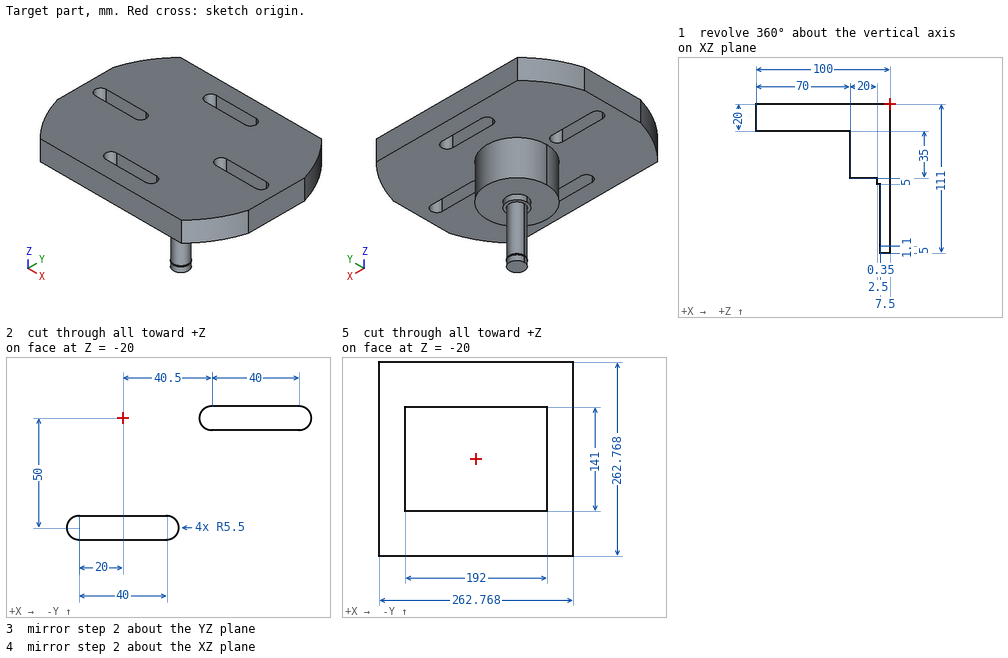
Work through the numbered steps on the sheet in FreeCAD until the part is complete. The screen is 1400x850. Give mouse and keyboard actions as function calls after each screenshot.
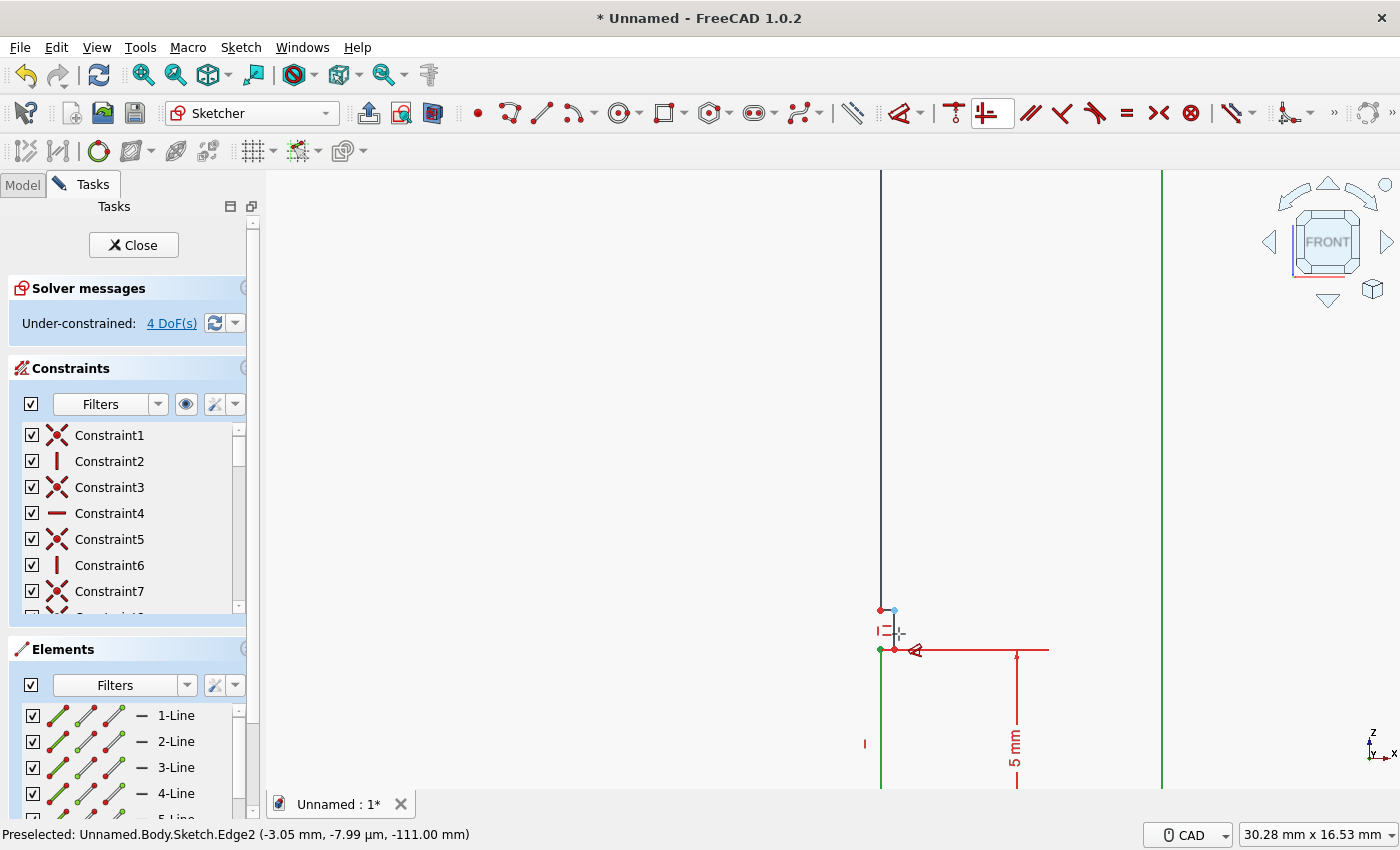
click(894, 630)
click(928, 630)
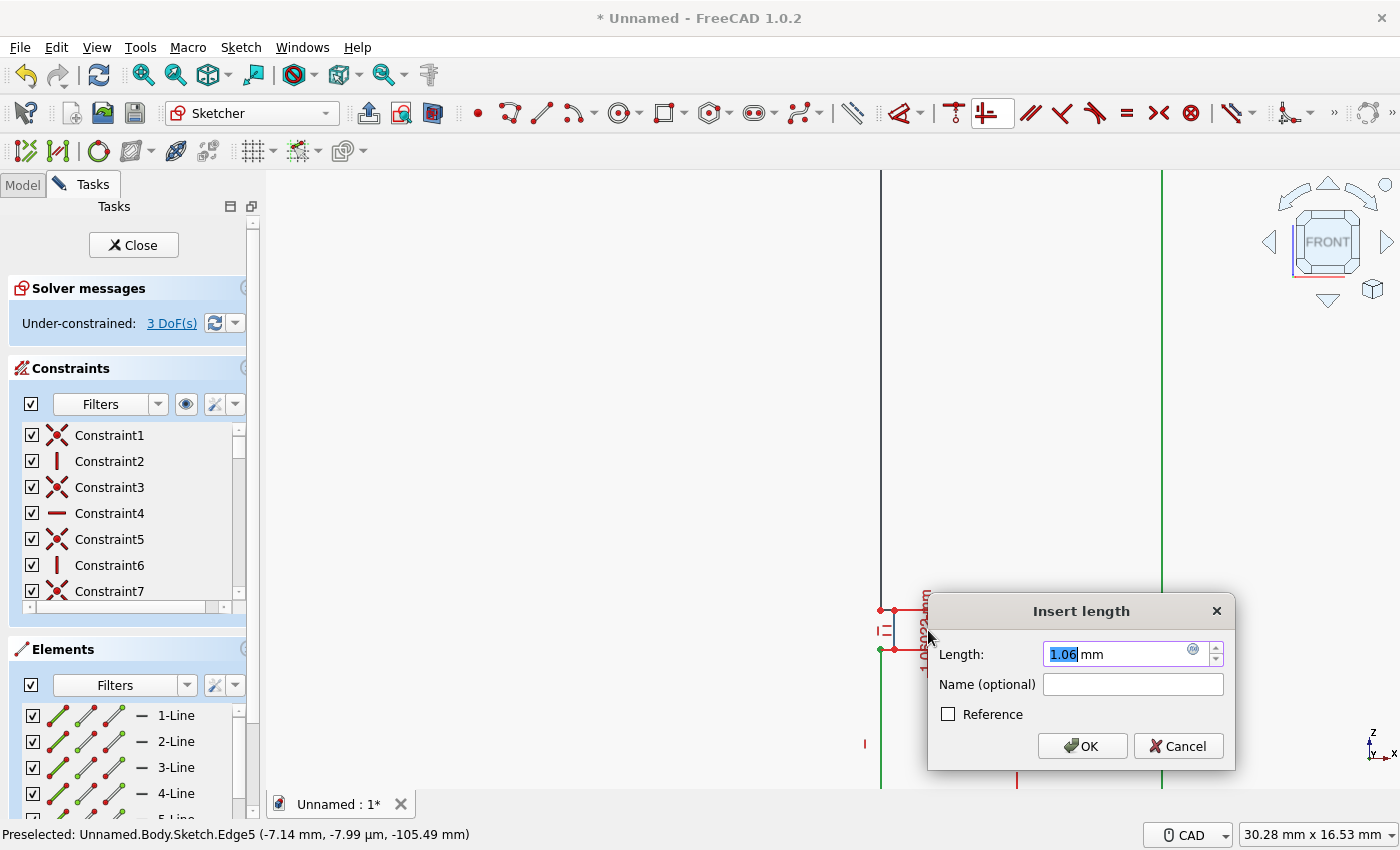
text(1.1)
key(Return)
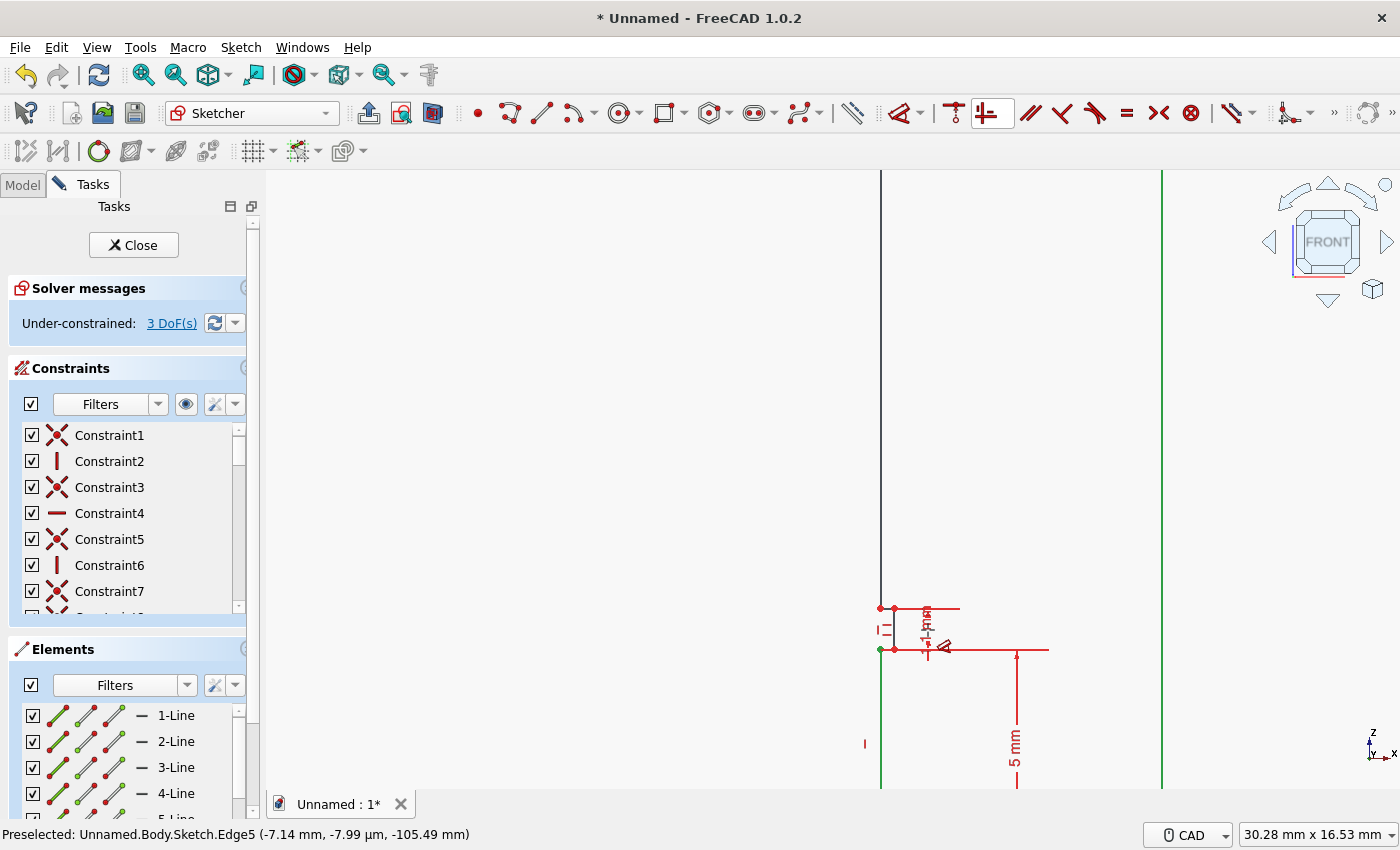
scroll(912, 651, down, 12)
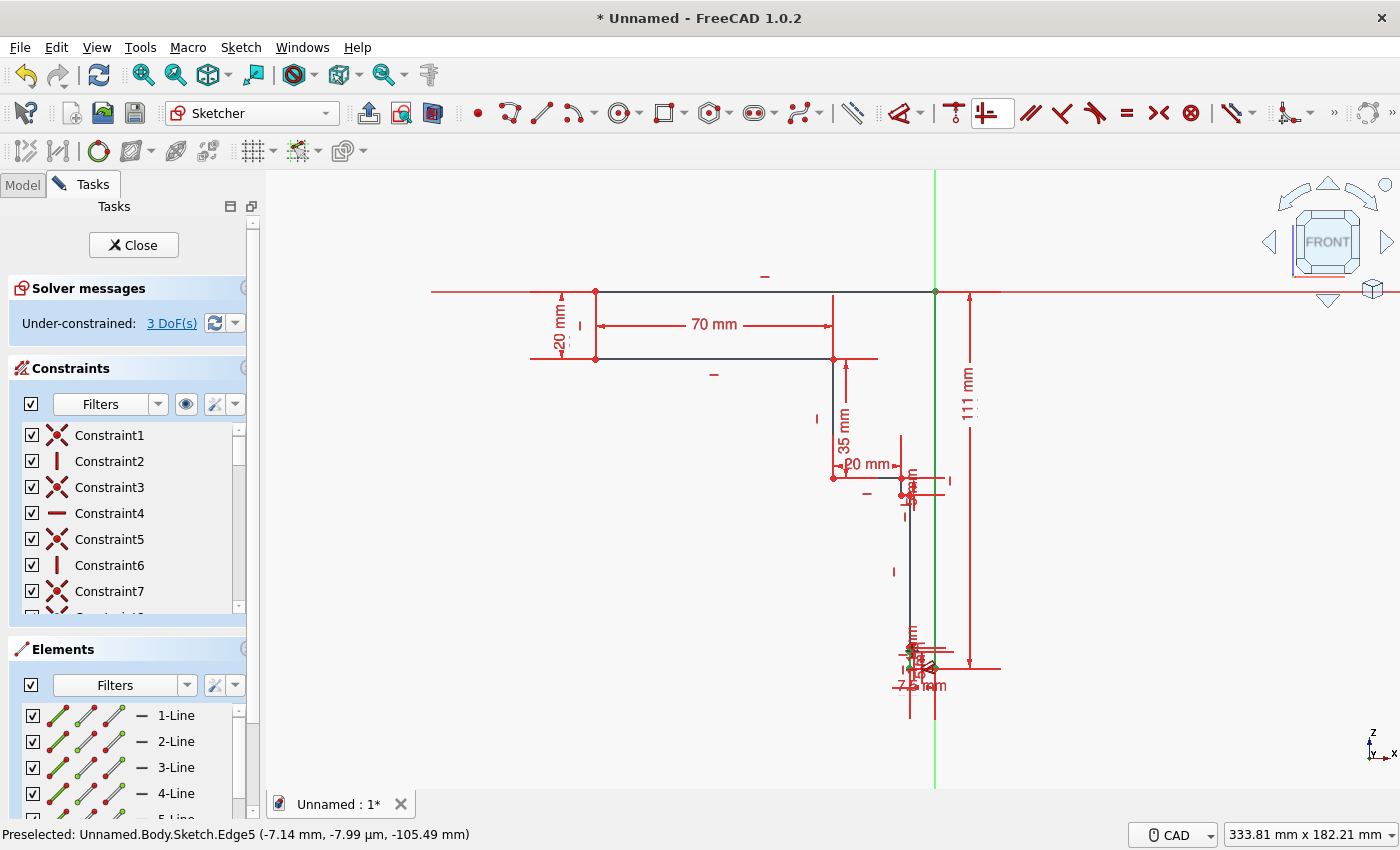
scroll(907, 495, up, 9)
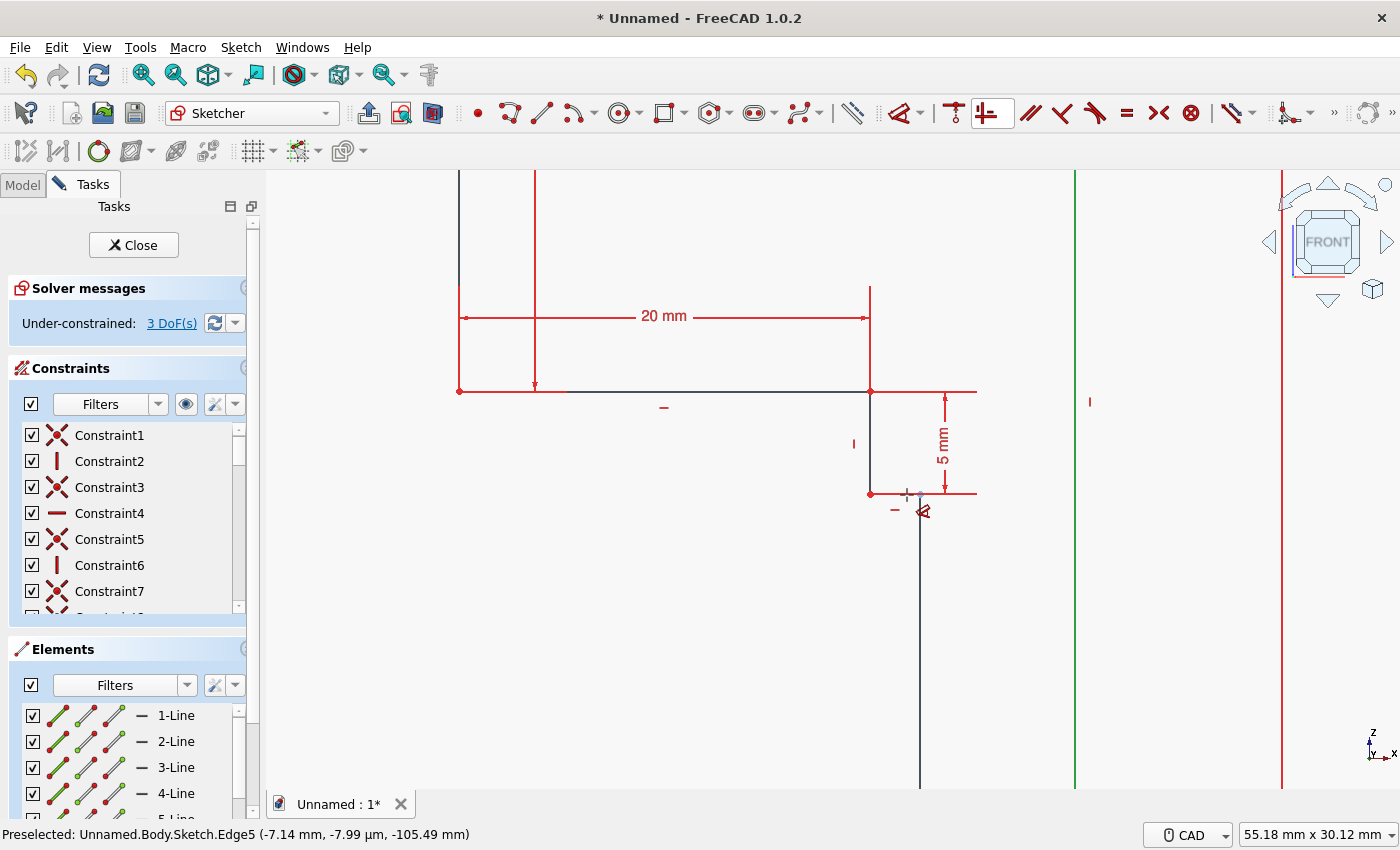
click(905, 494)
click(895, 528)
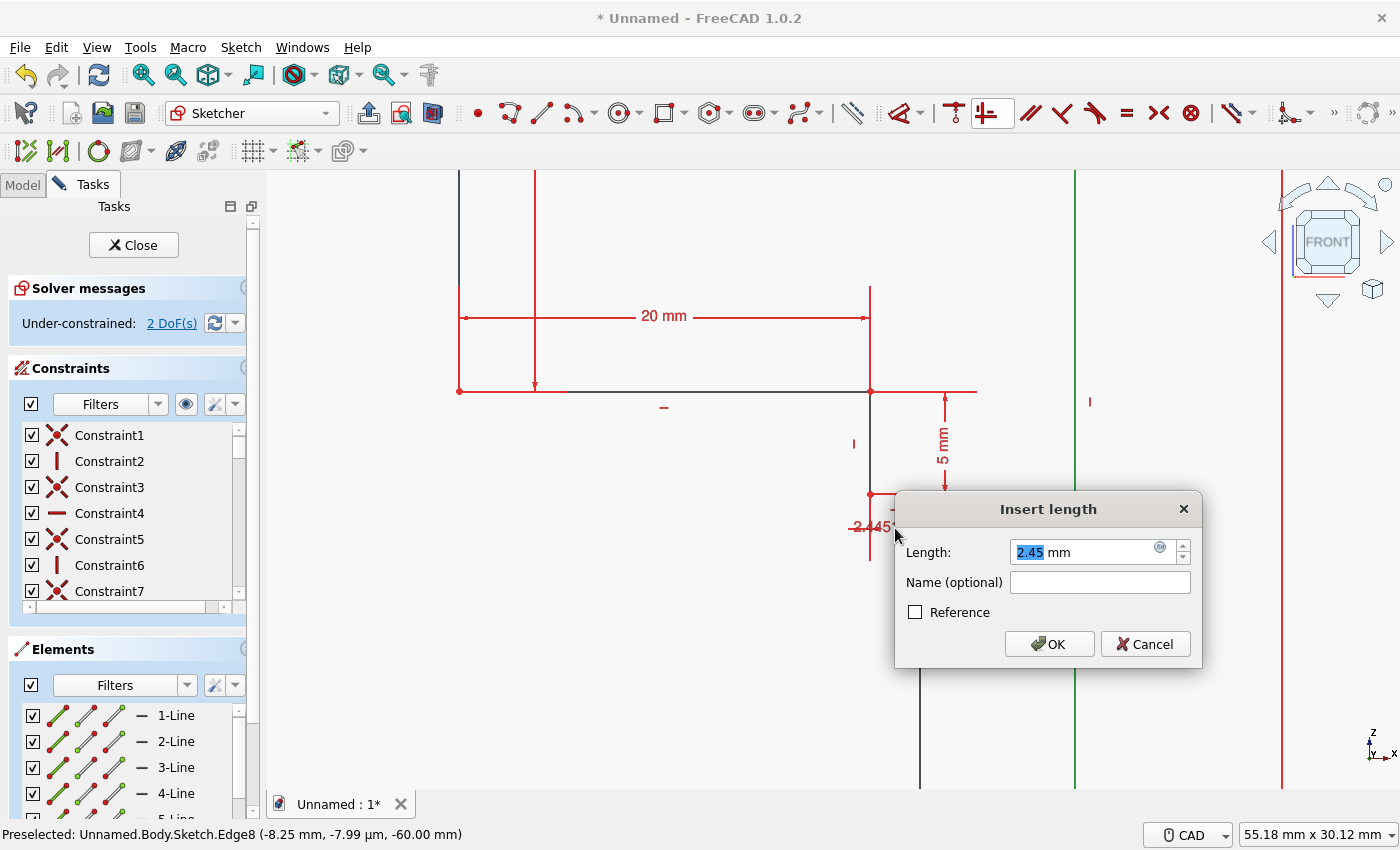
text(2.5)
key(Return)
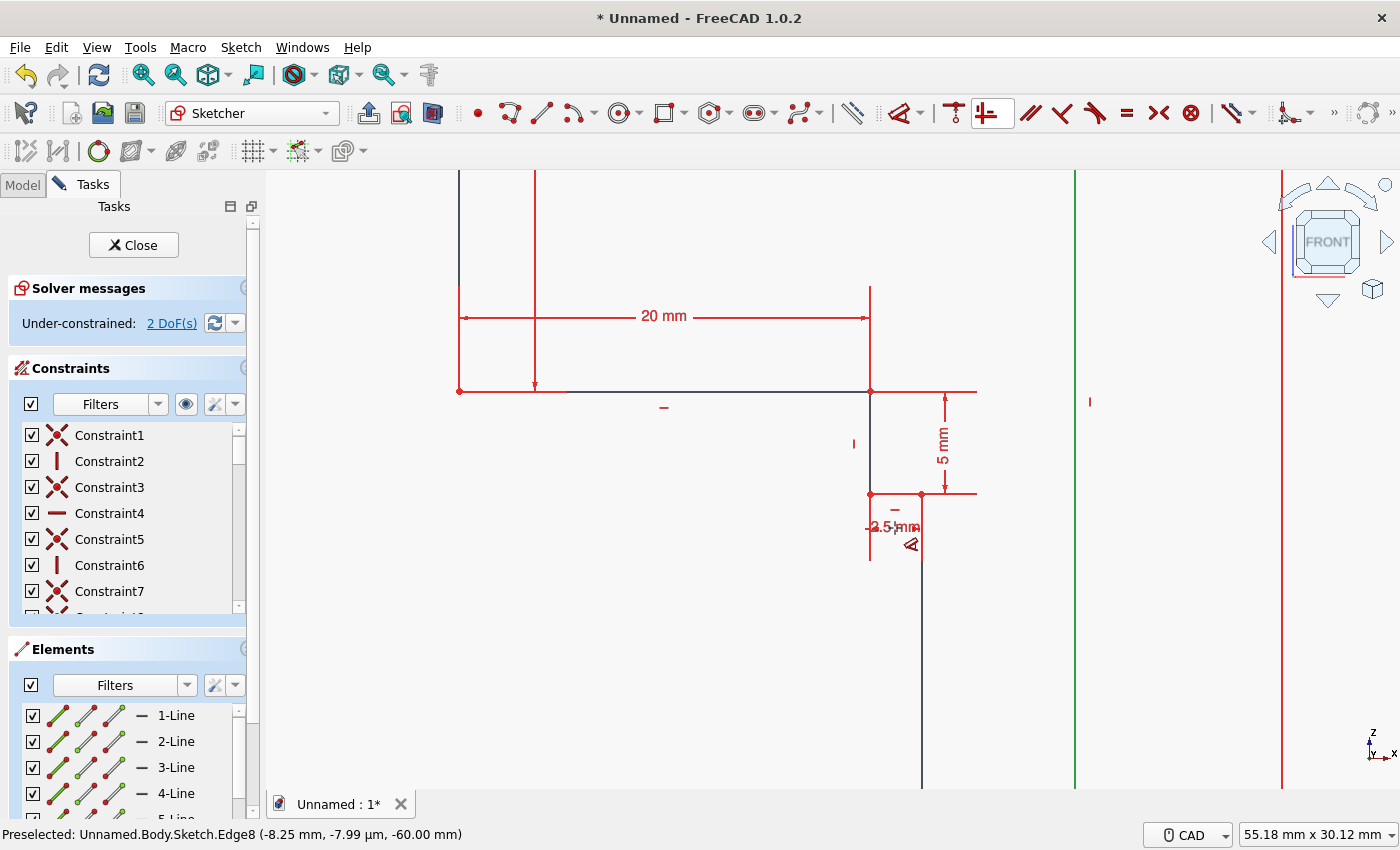
scroll(907, 495, down, 9)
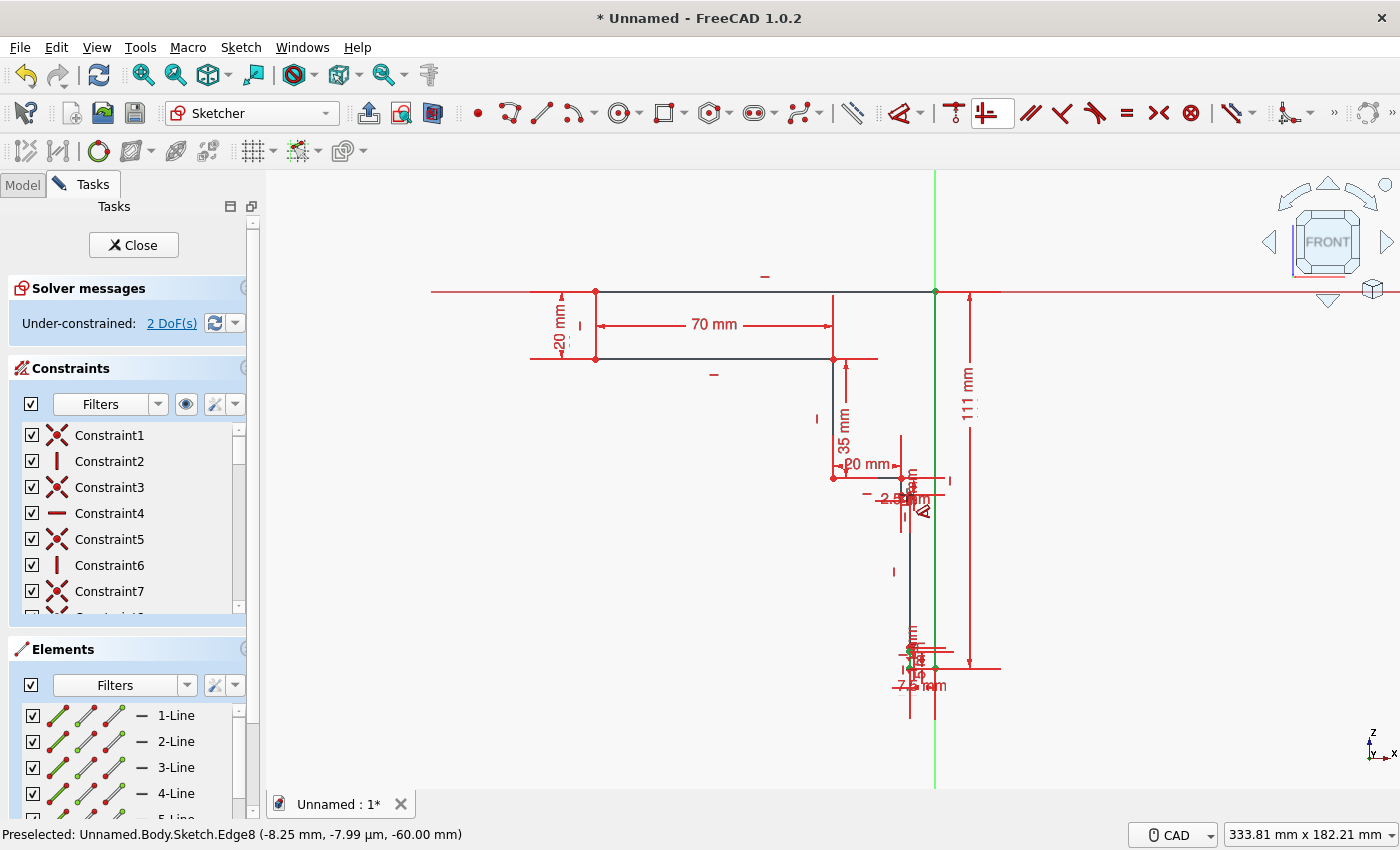
click(698, 292)
click(765, 258)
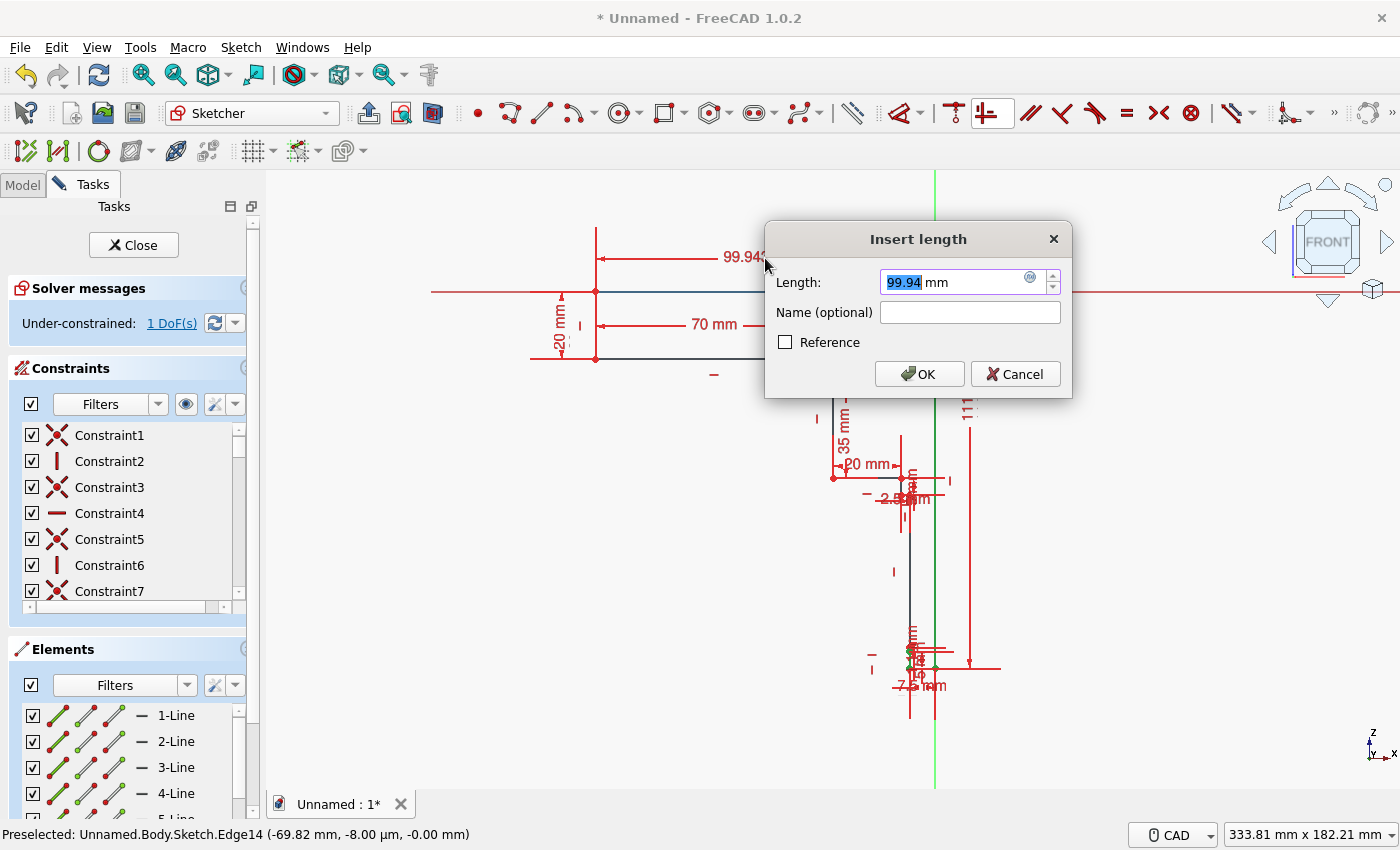
text(100)
key(Return)